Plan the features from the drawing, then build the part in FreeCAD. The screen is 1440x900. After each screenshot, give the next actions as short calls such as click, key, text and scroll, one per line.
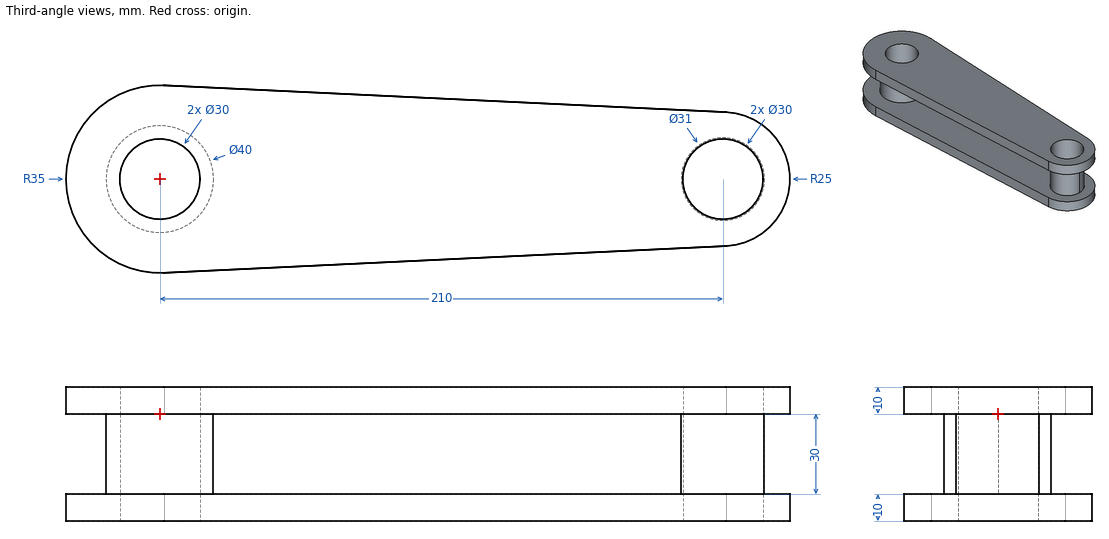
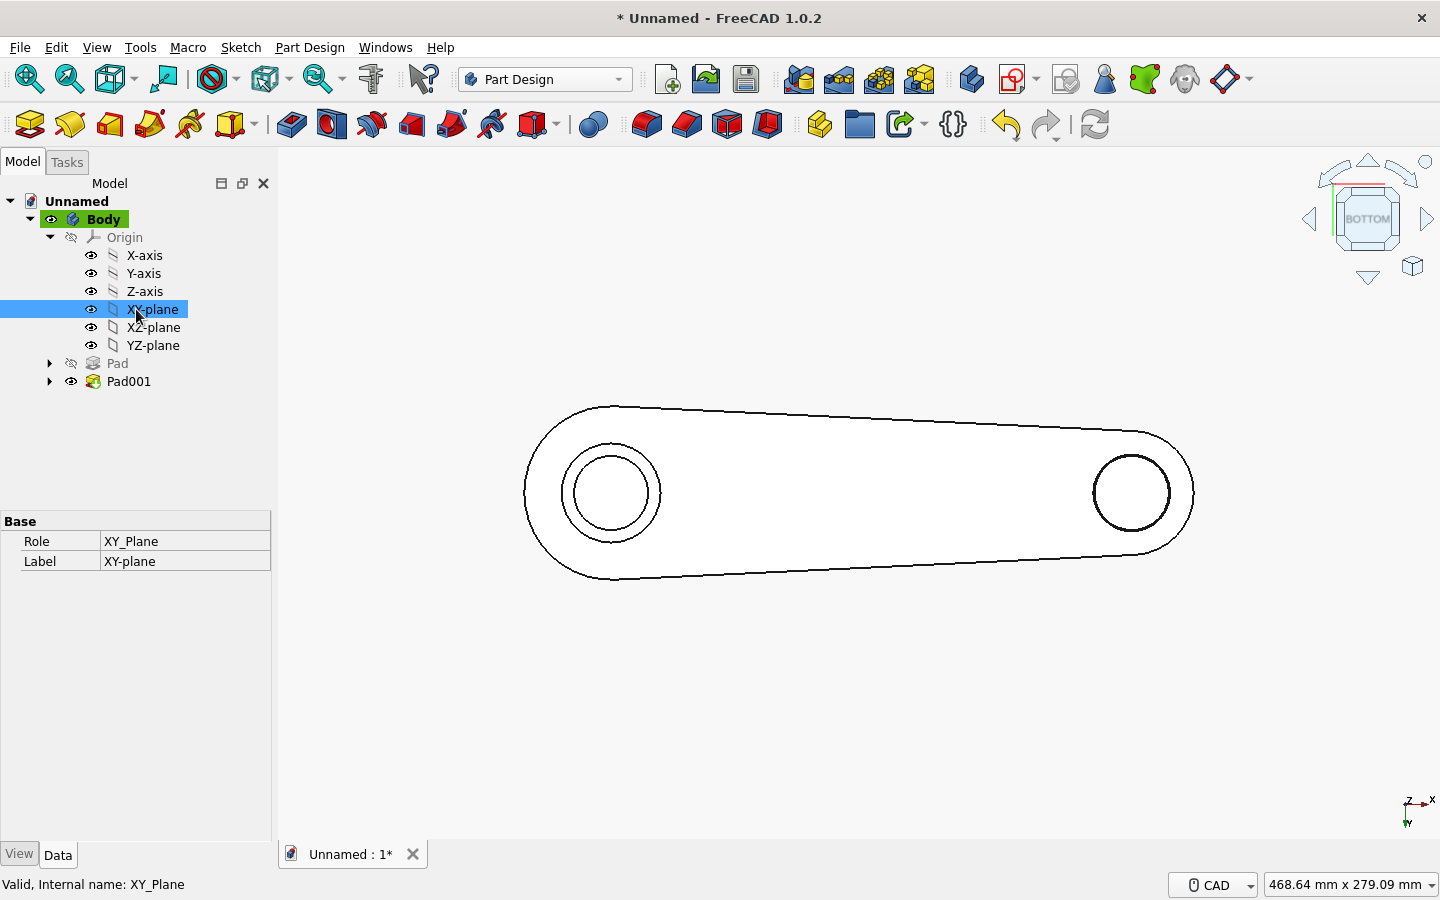
click(1226, 80)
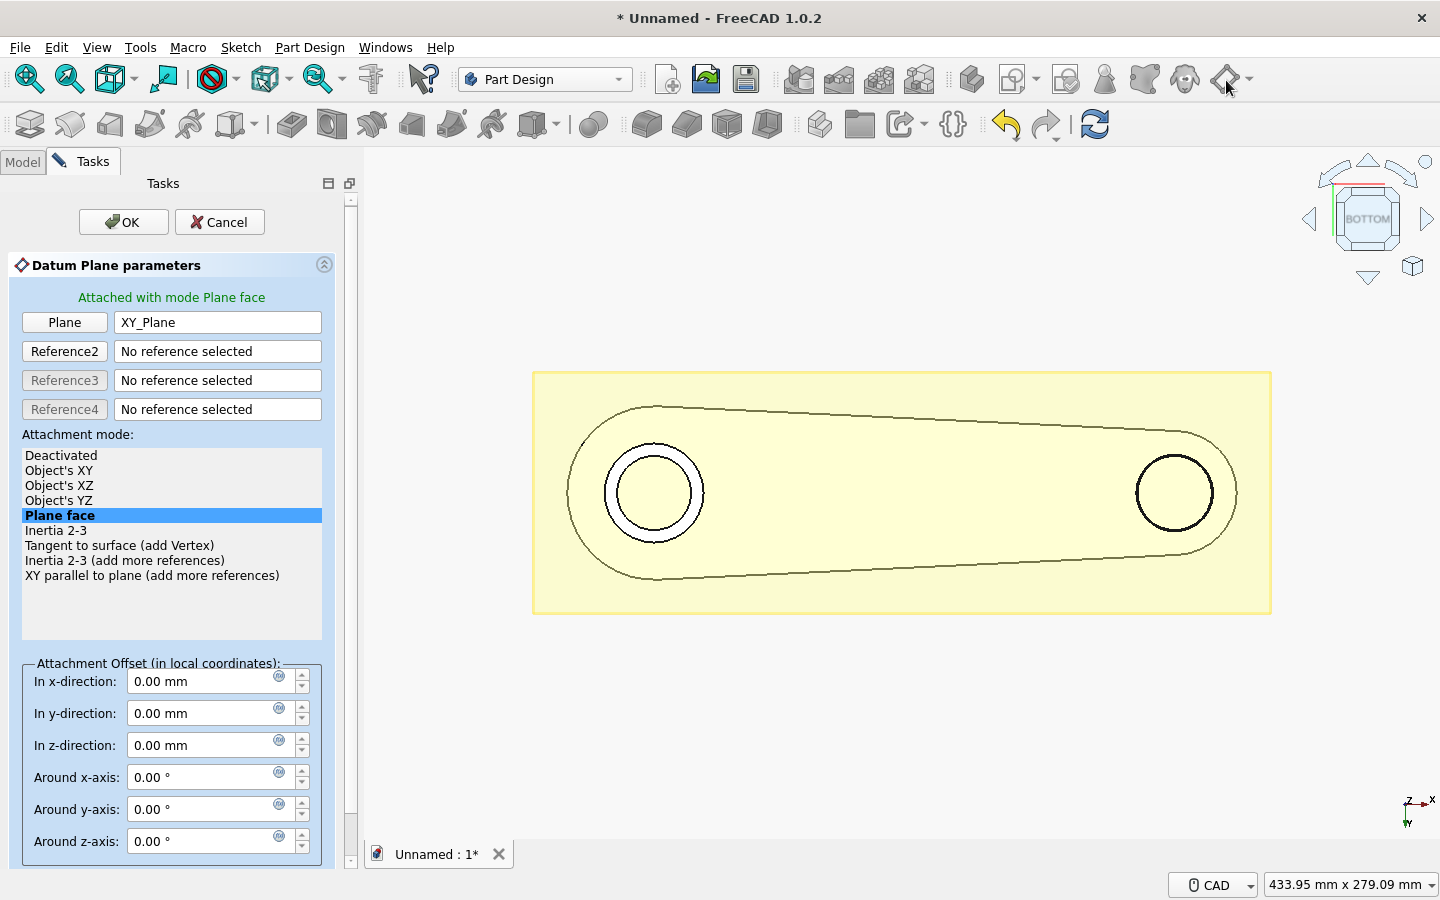
triple_click(210, 745)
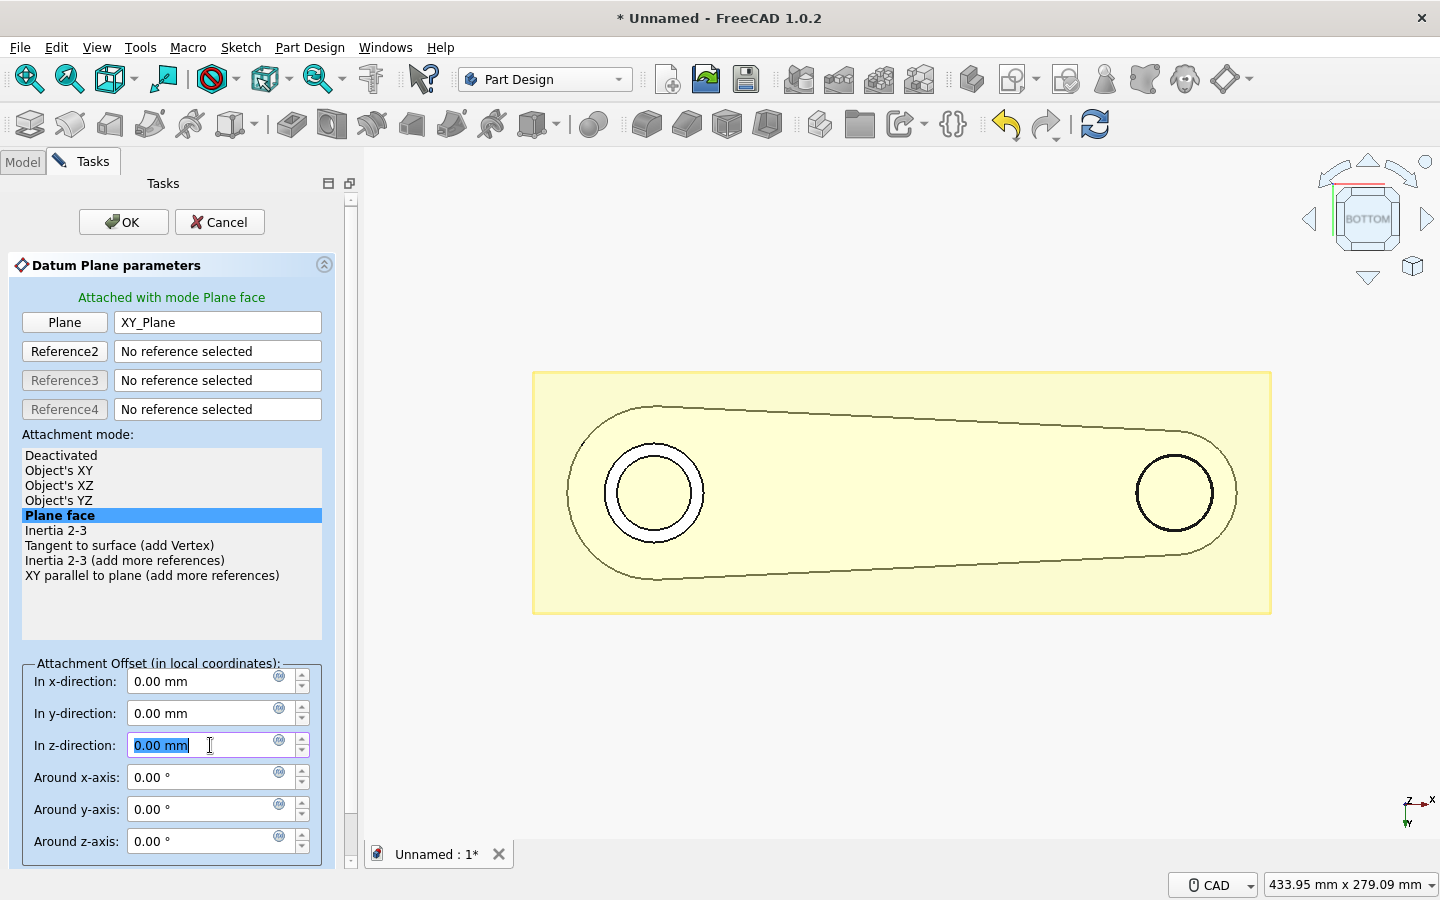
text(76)
key(Tab)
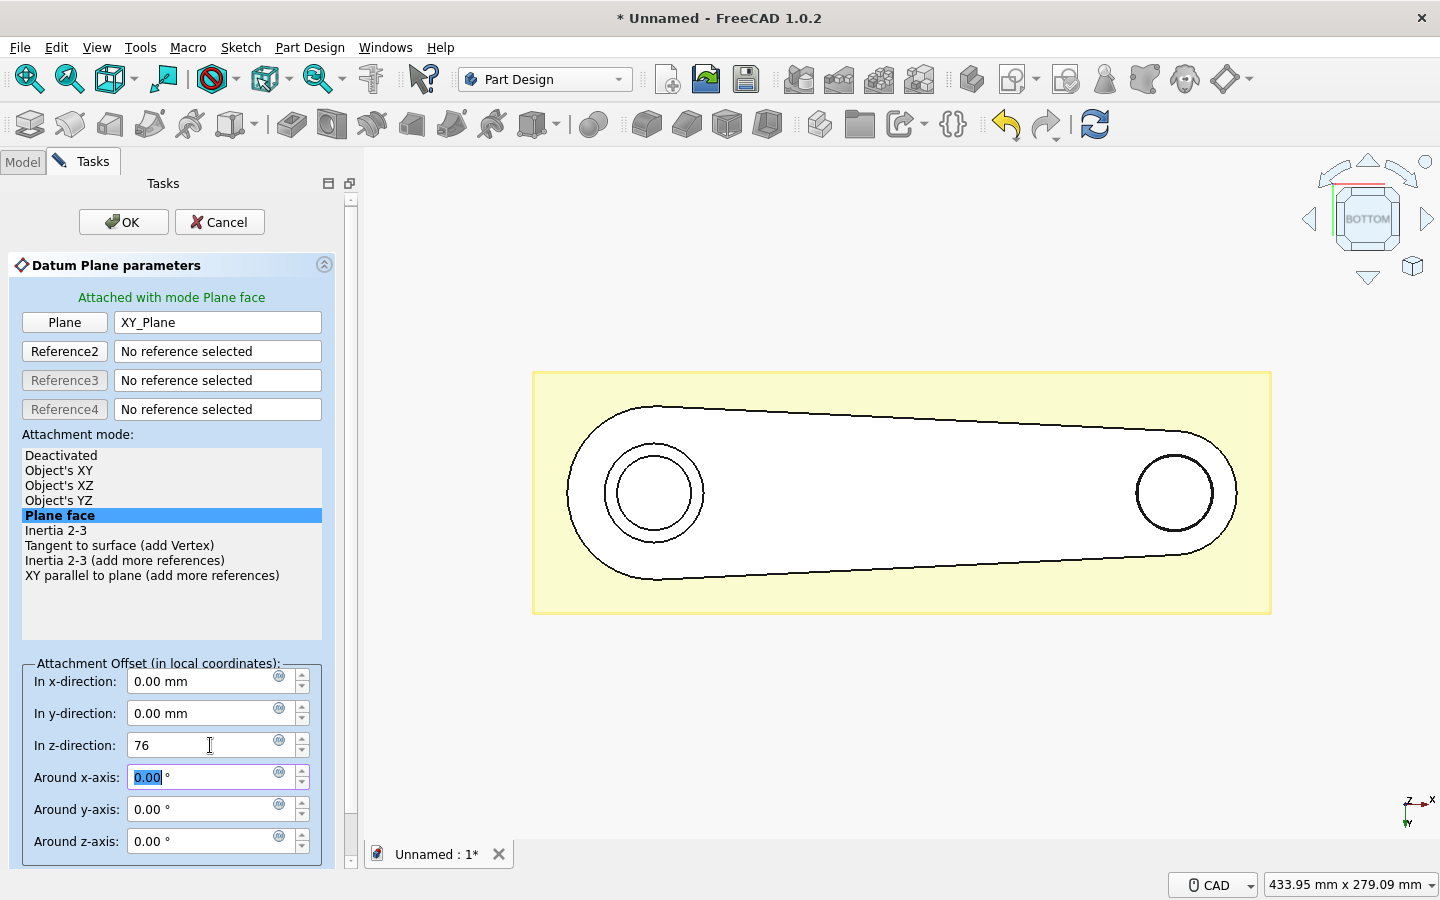
click(124, 222)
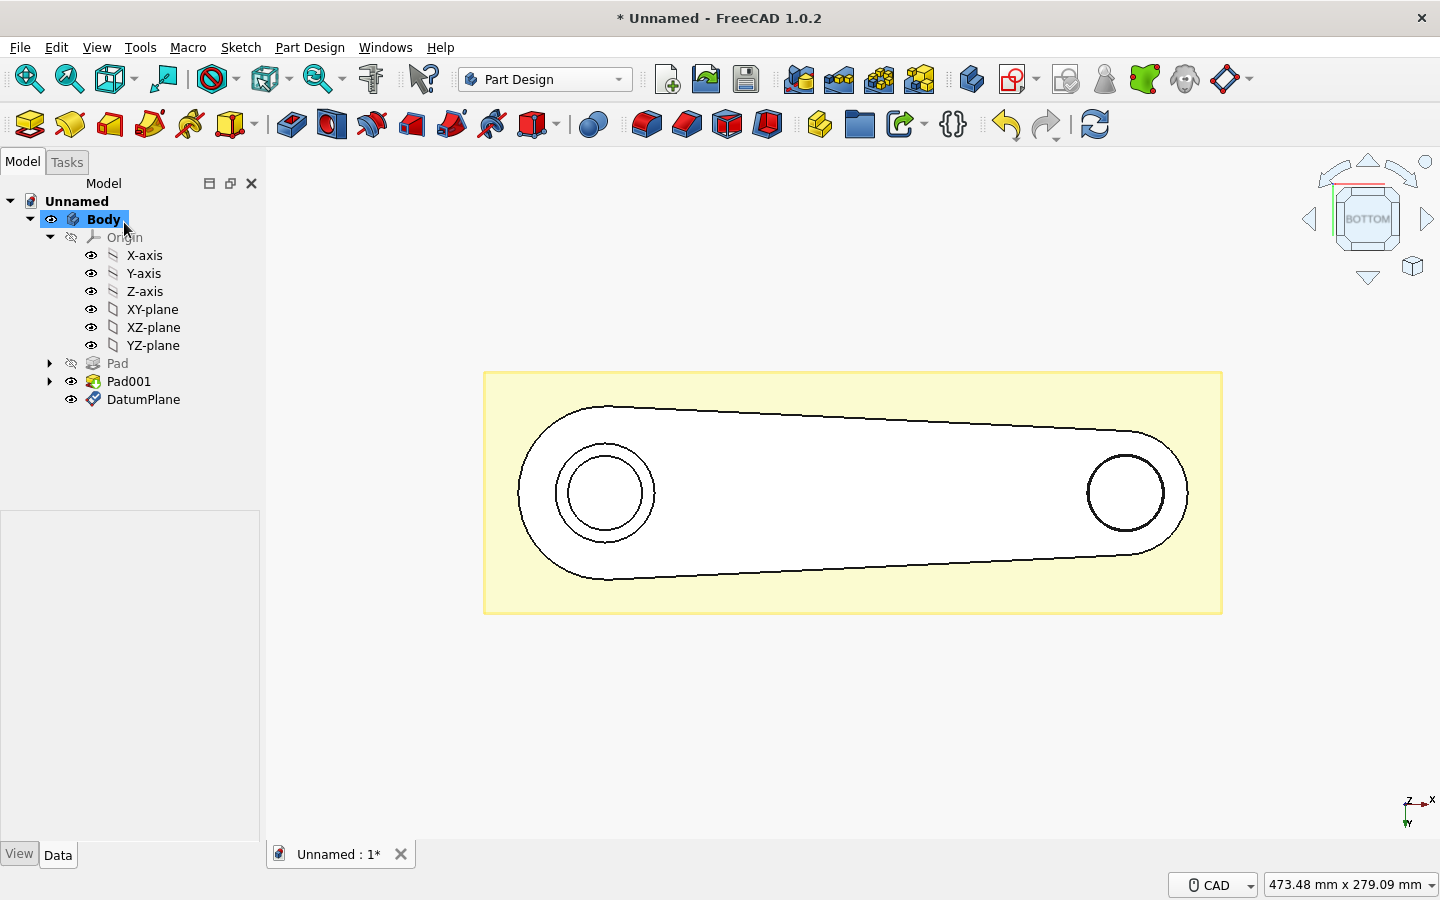
click(116, 399)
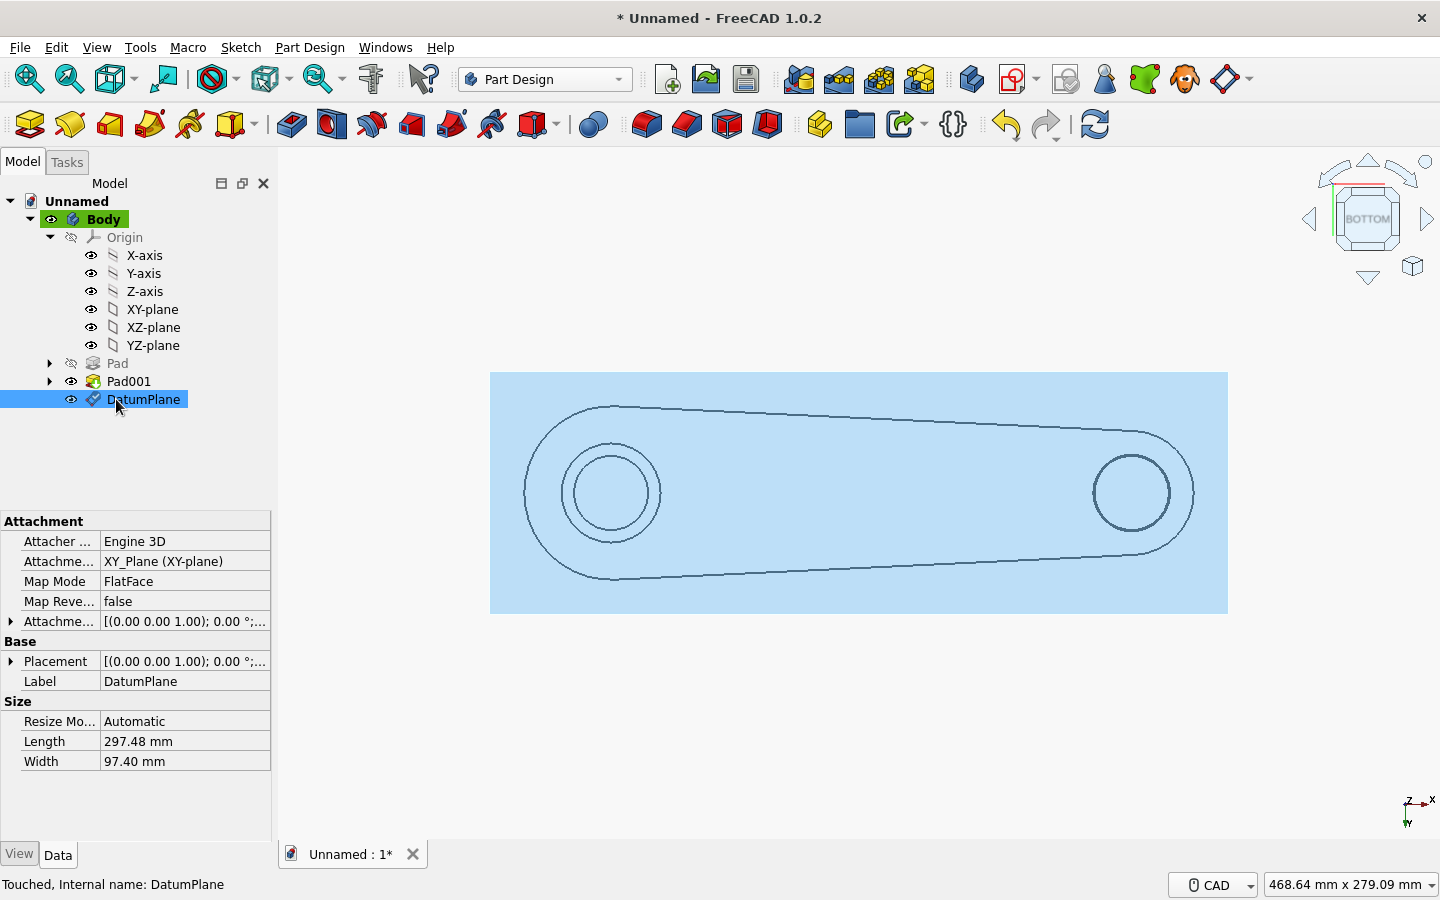
click(1012, 80)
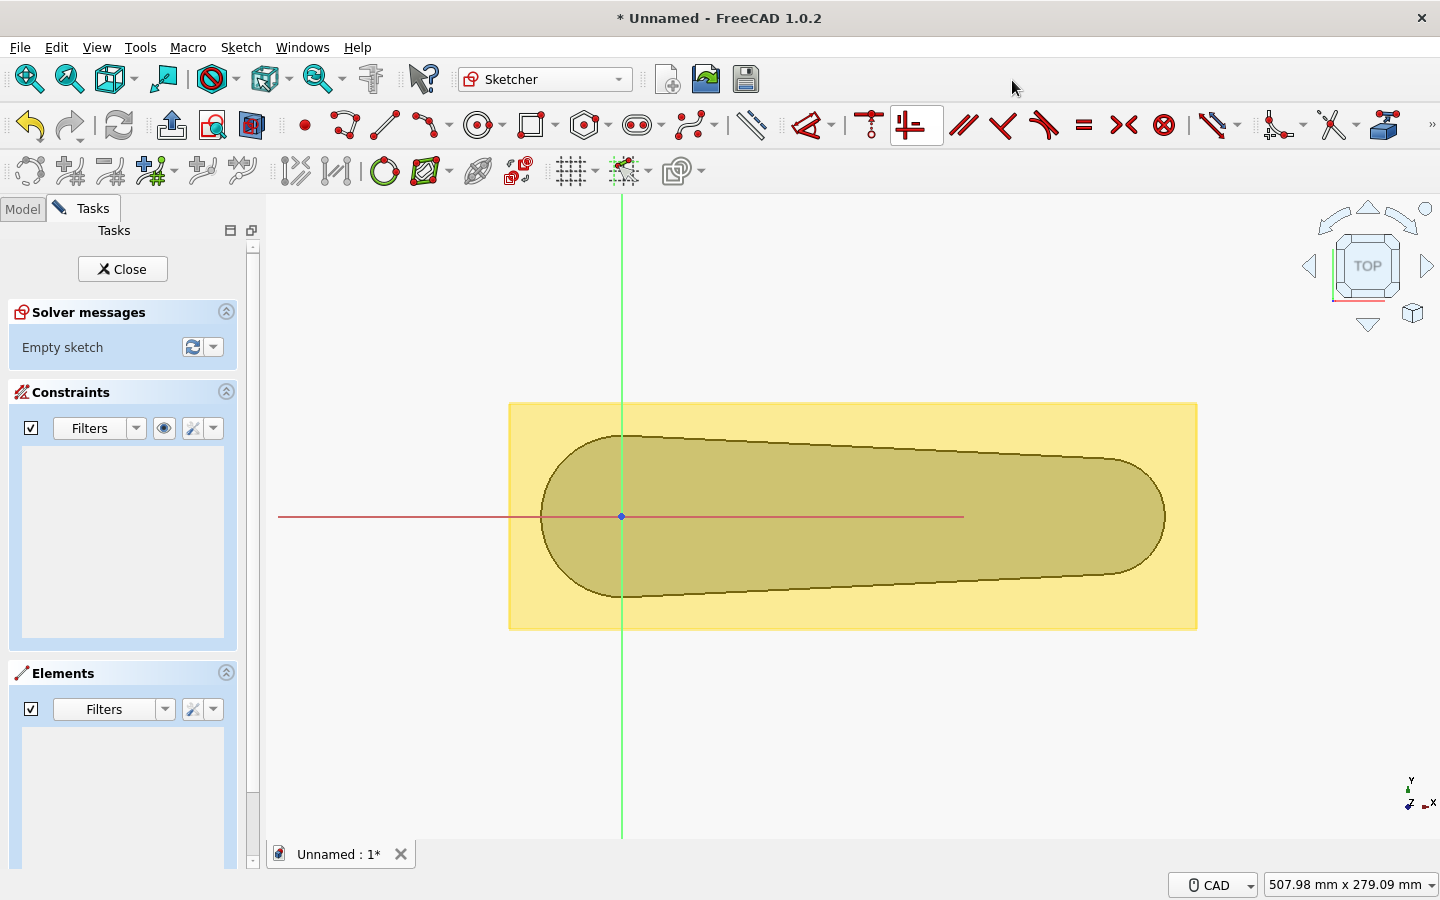
click(478, 126)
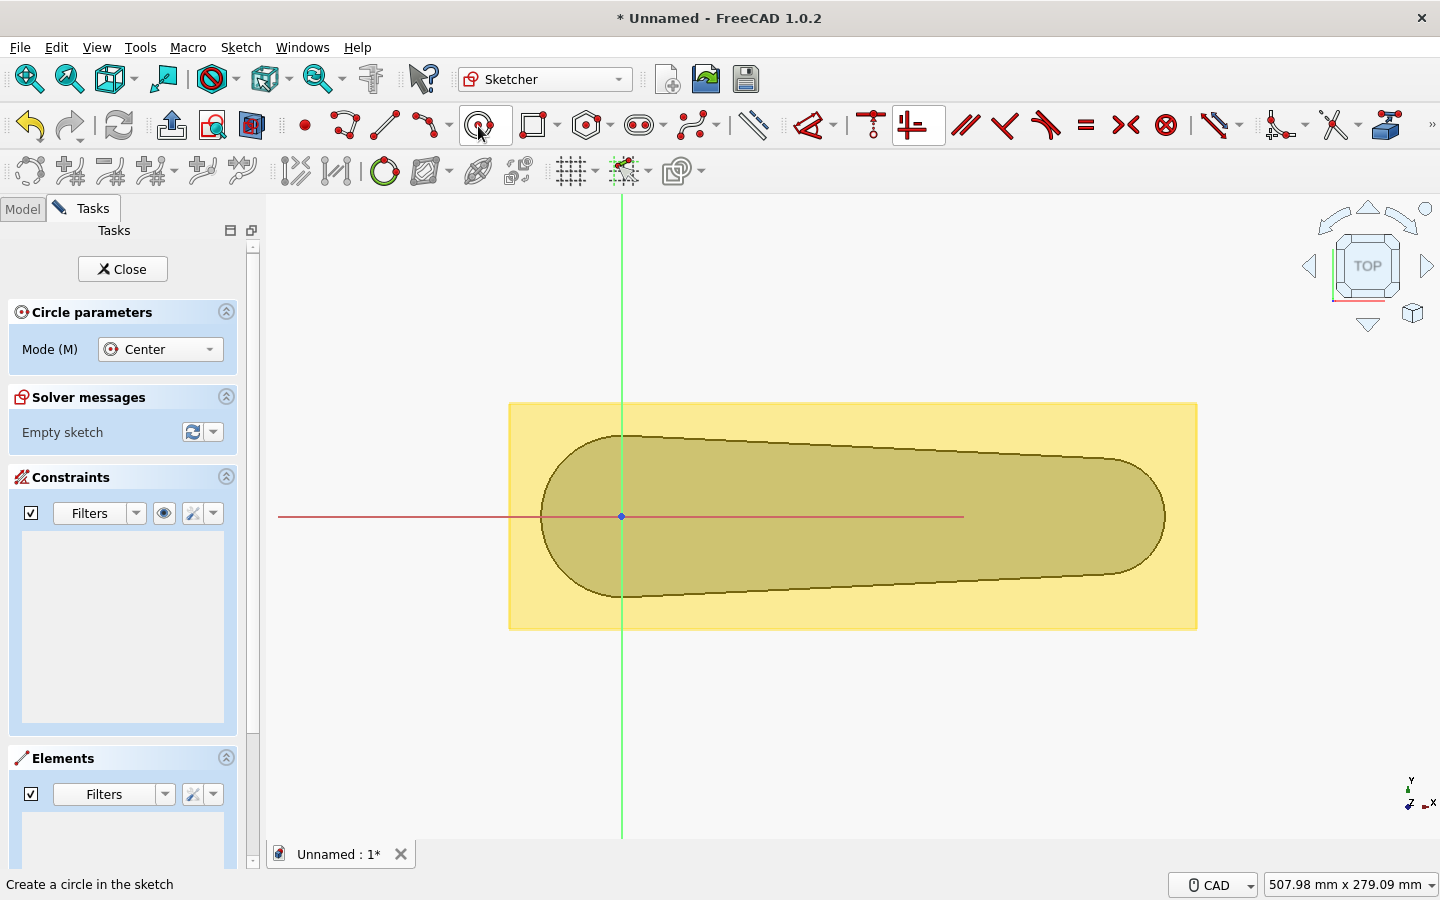
click(622, 516)
move(646, 492)